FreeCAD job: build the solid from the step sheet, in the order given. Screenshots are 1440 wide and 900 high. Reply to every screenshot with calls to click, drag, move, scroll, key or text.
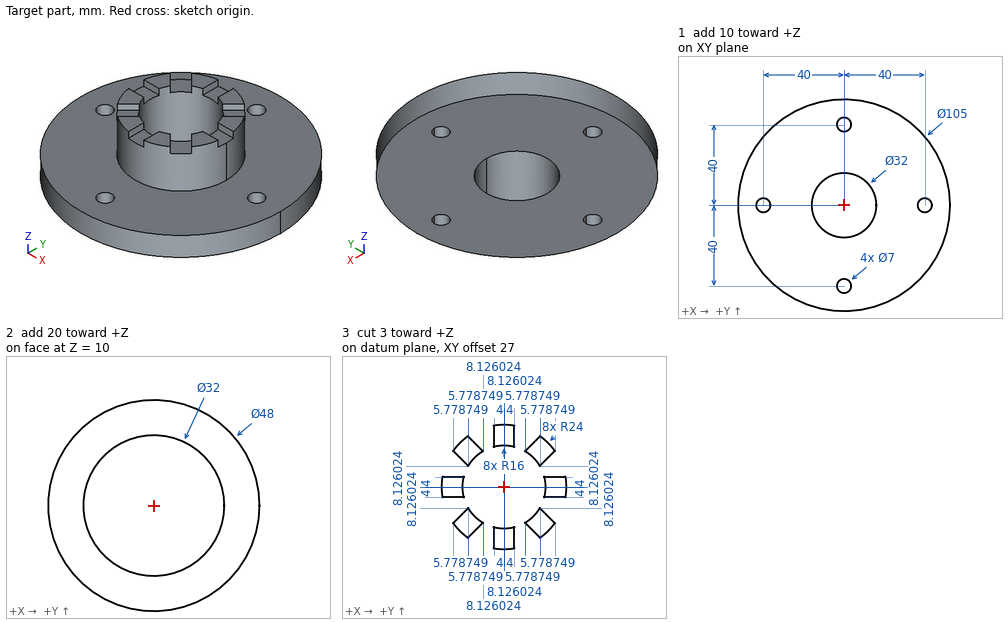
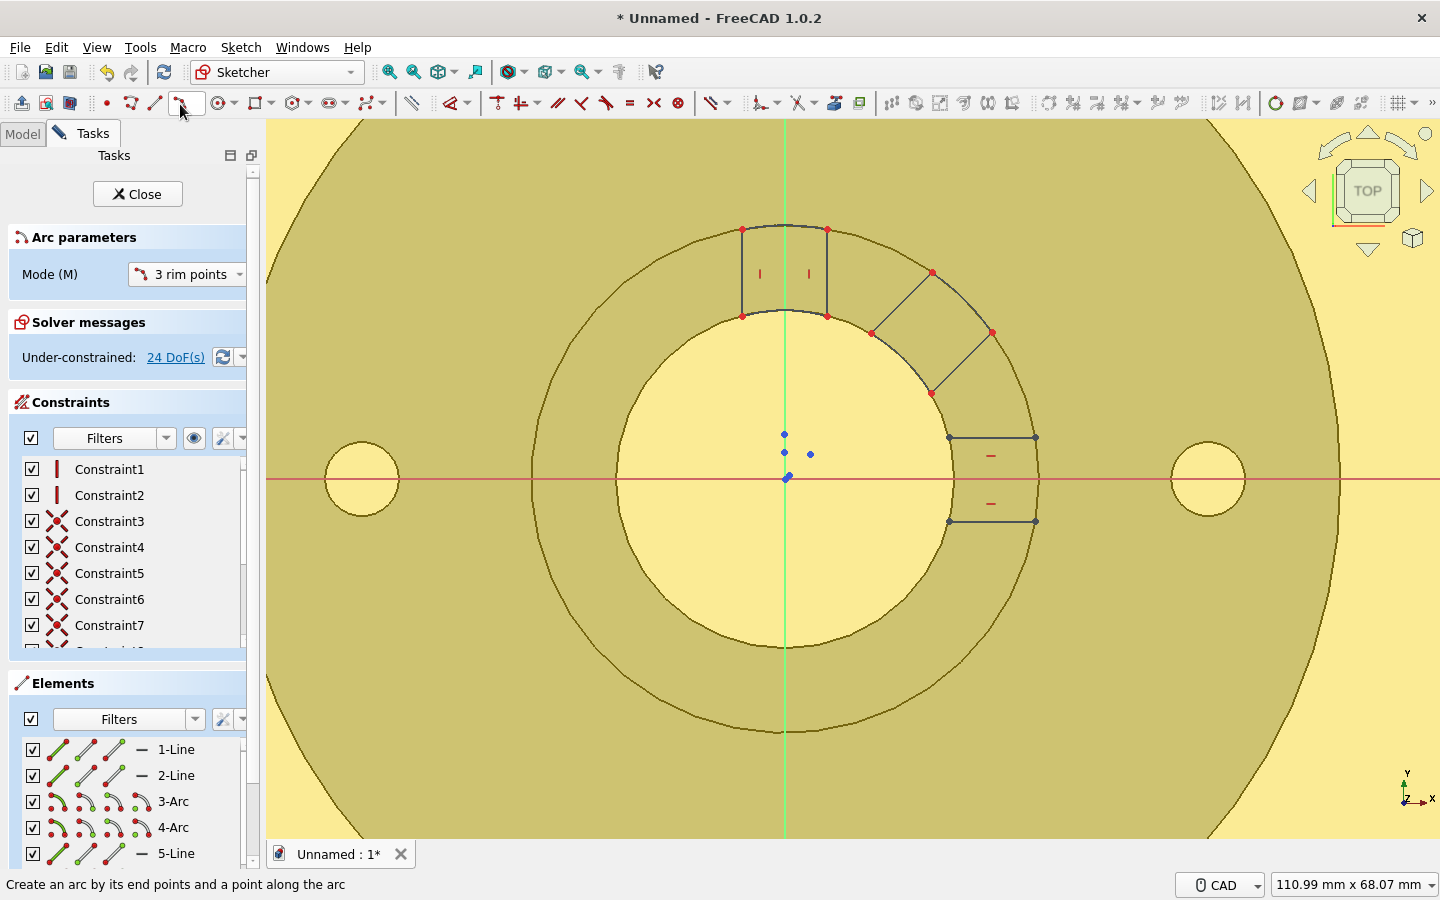
click(949, 438)
click(949, 522)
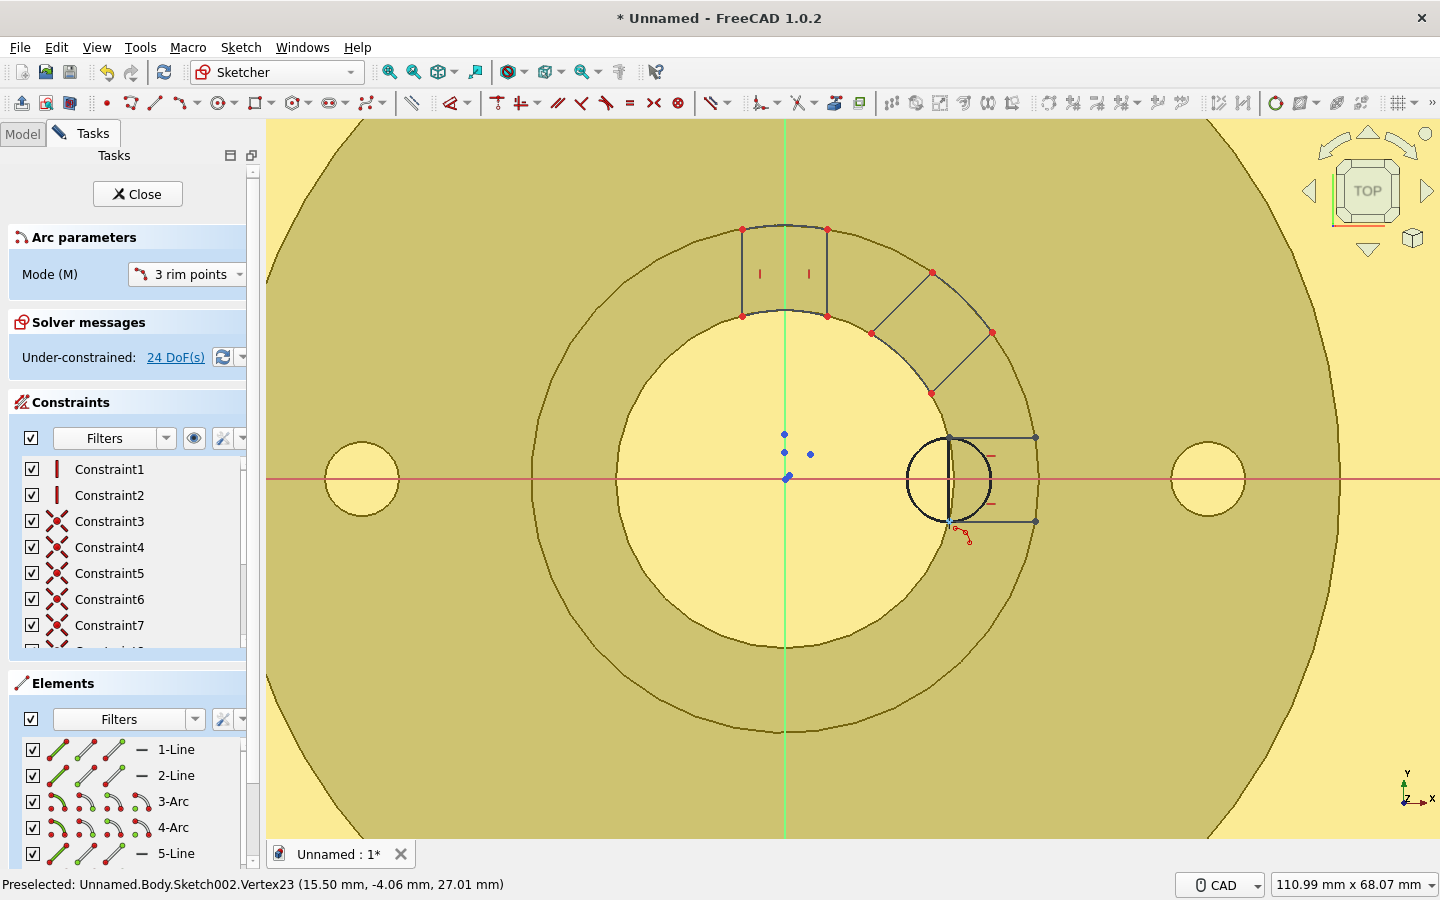
scroll(954, 488, up, 6)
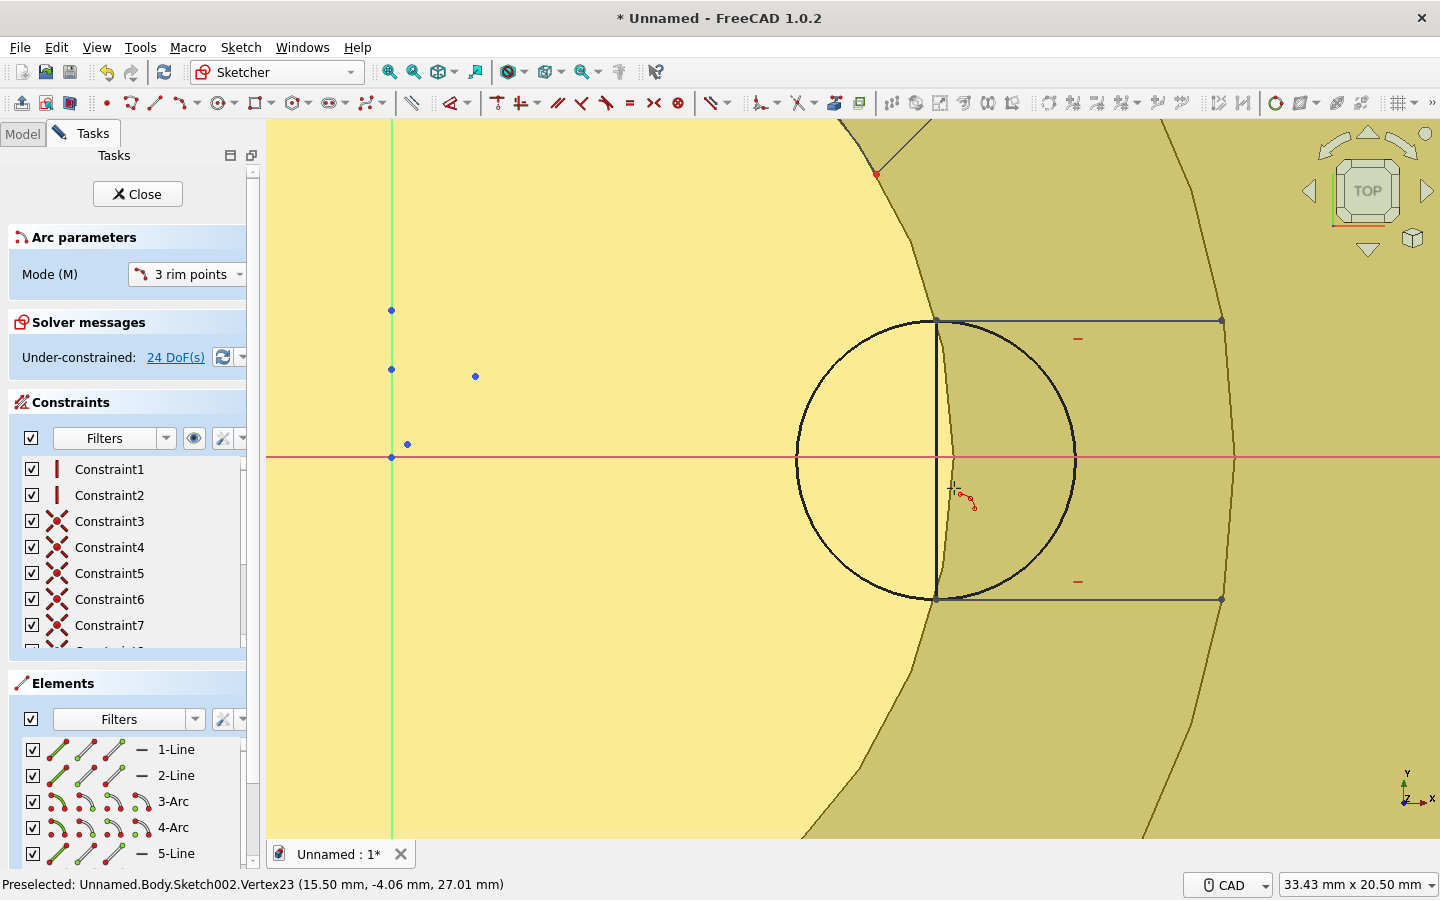
click(953, 486)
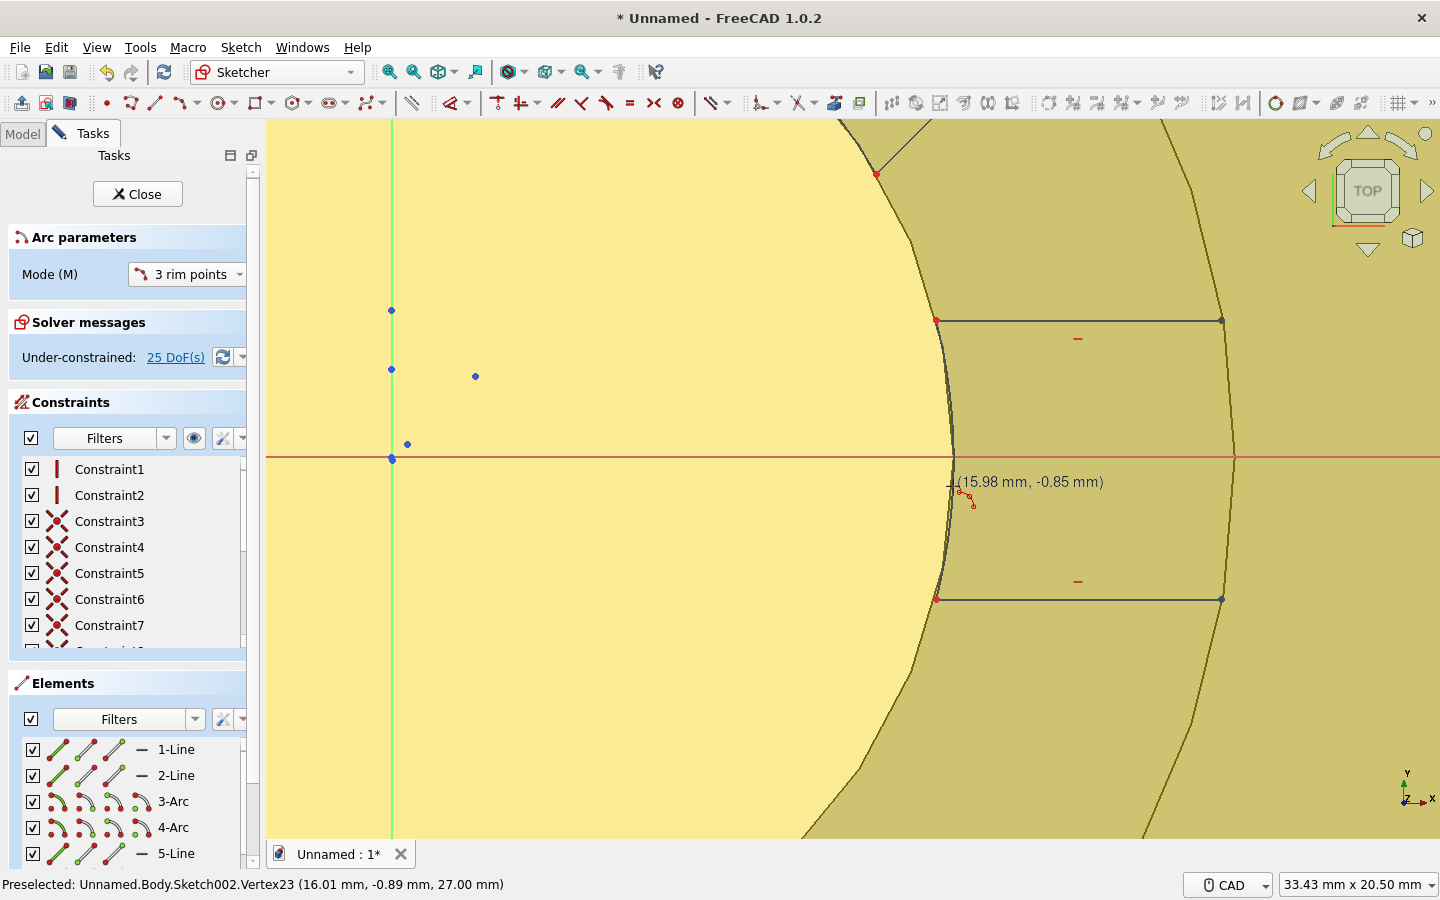
click(1222, 600)
click(1222, 321)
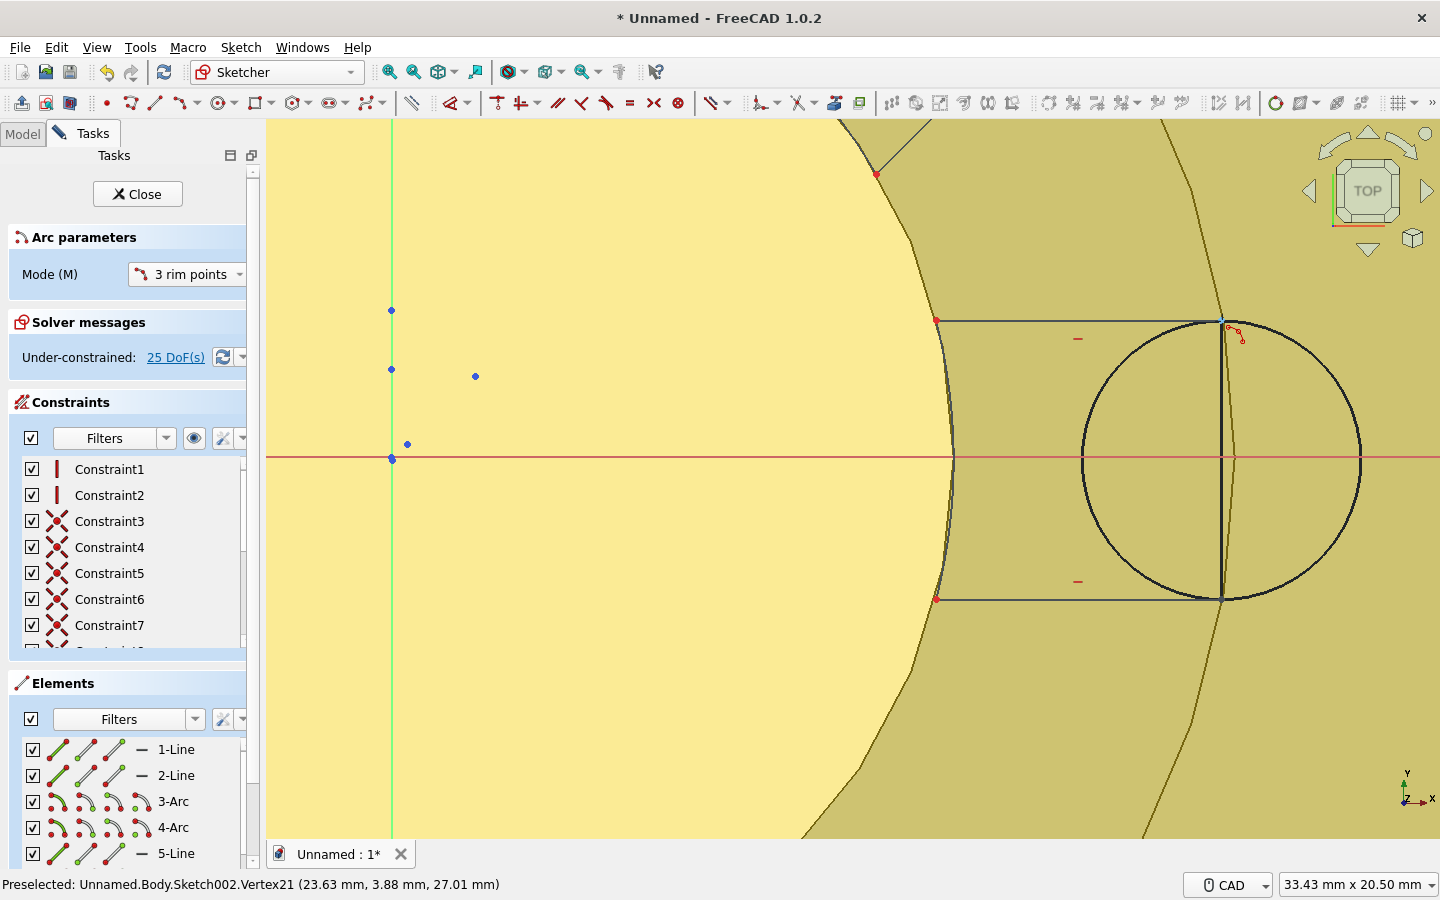
scroll(1234, 485, up, 2)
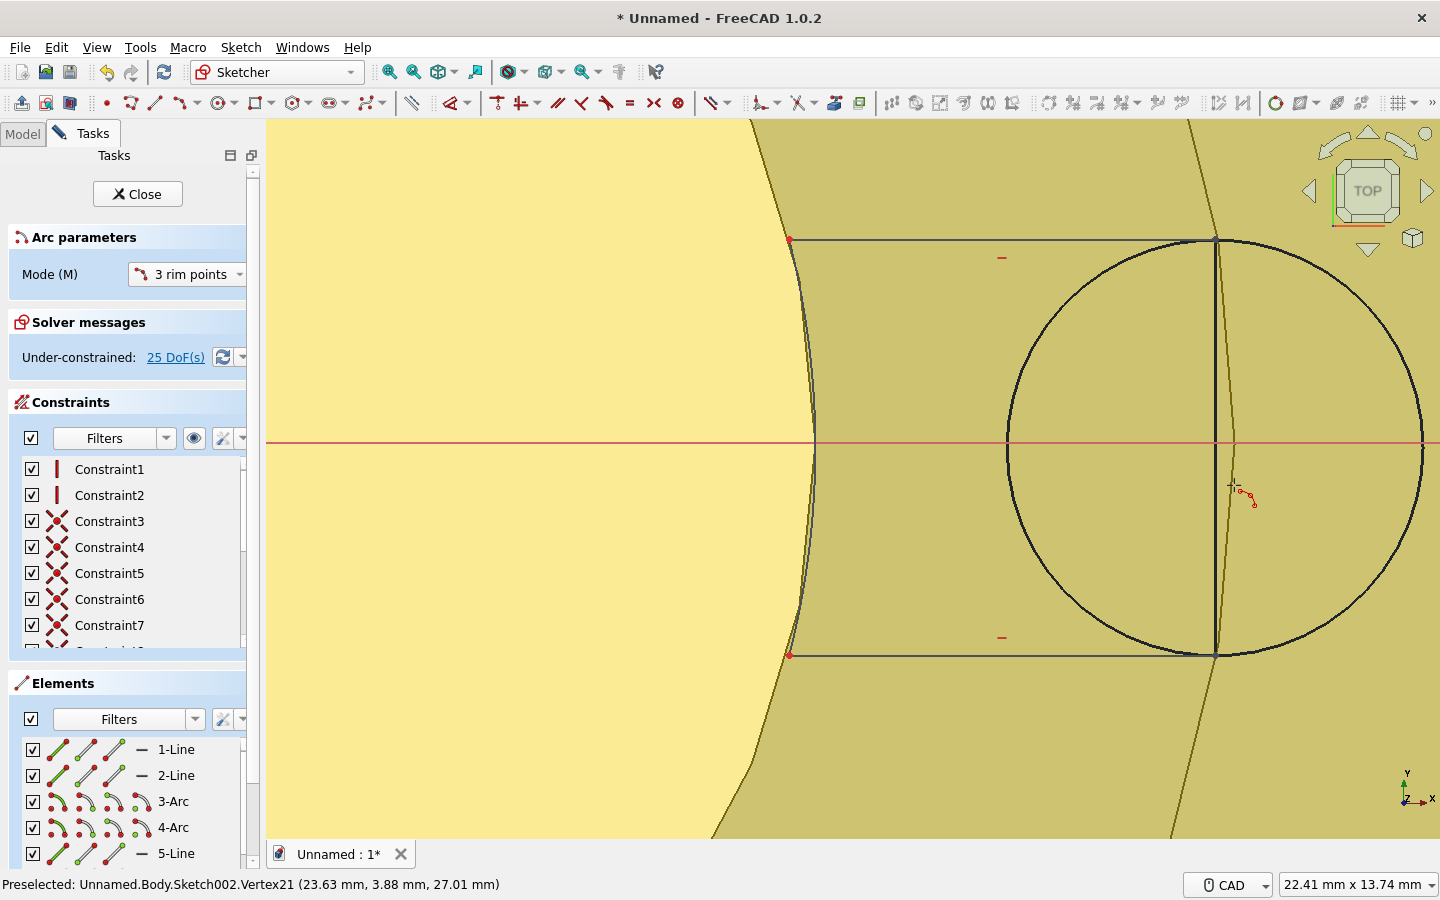
click(1234, 485)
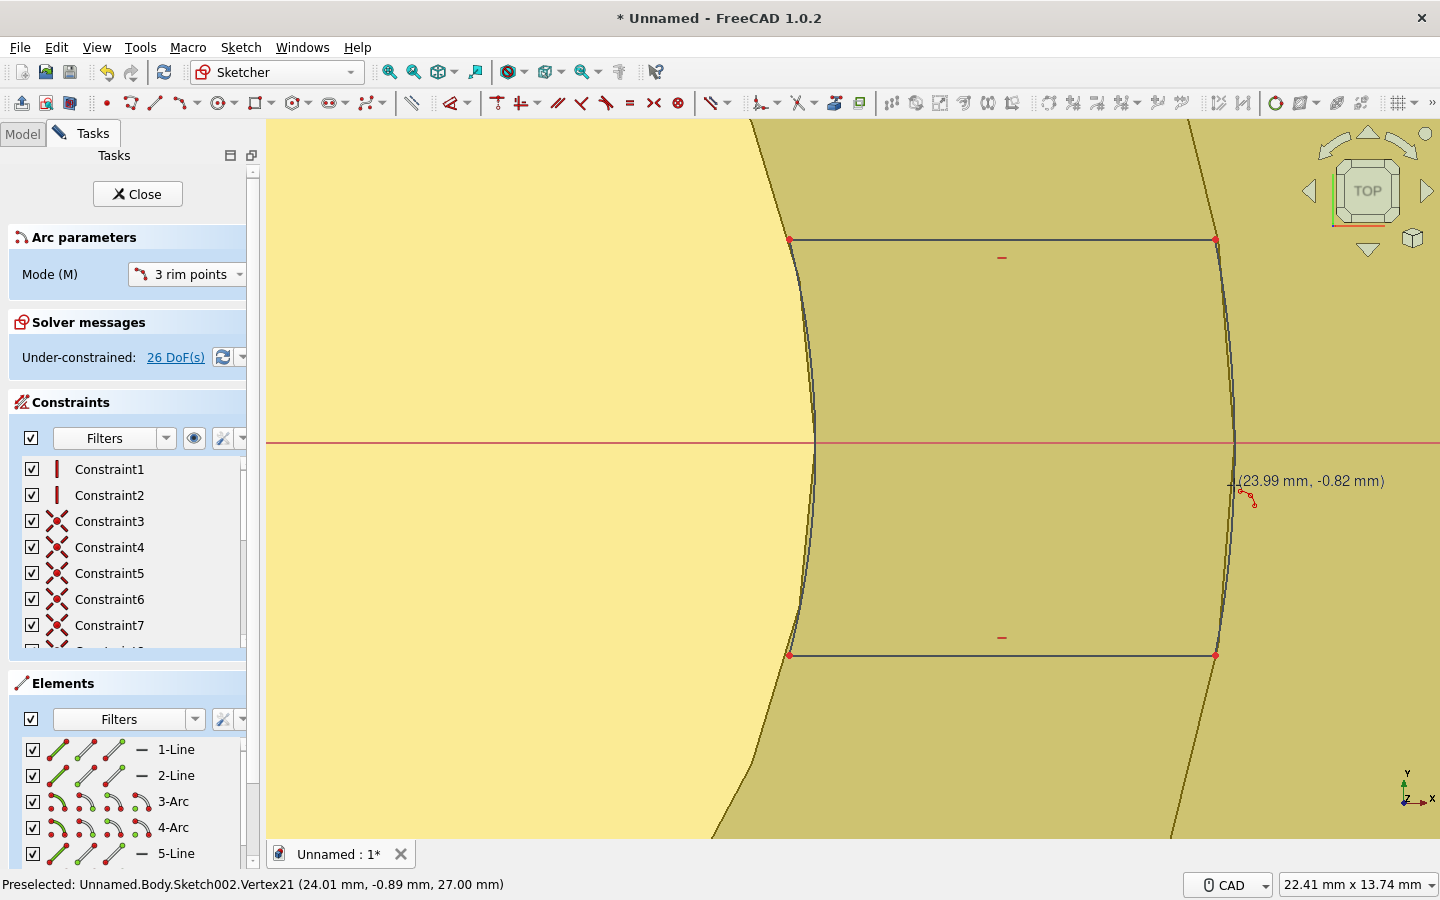
click(156, 104)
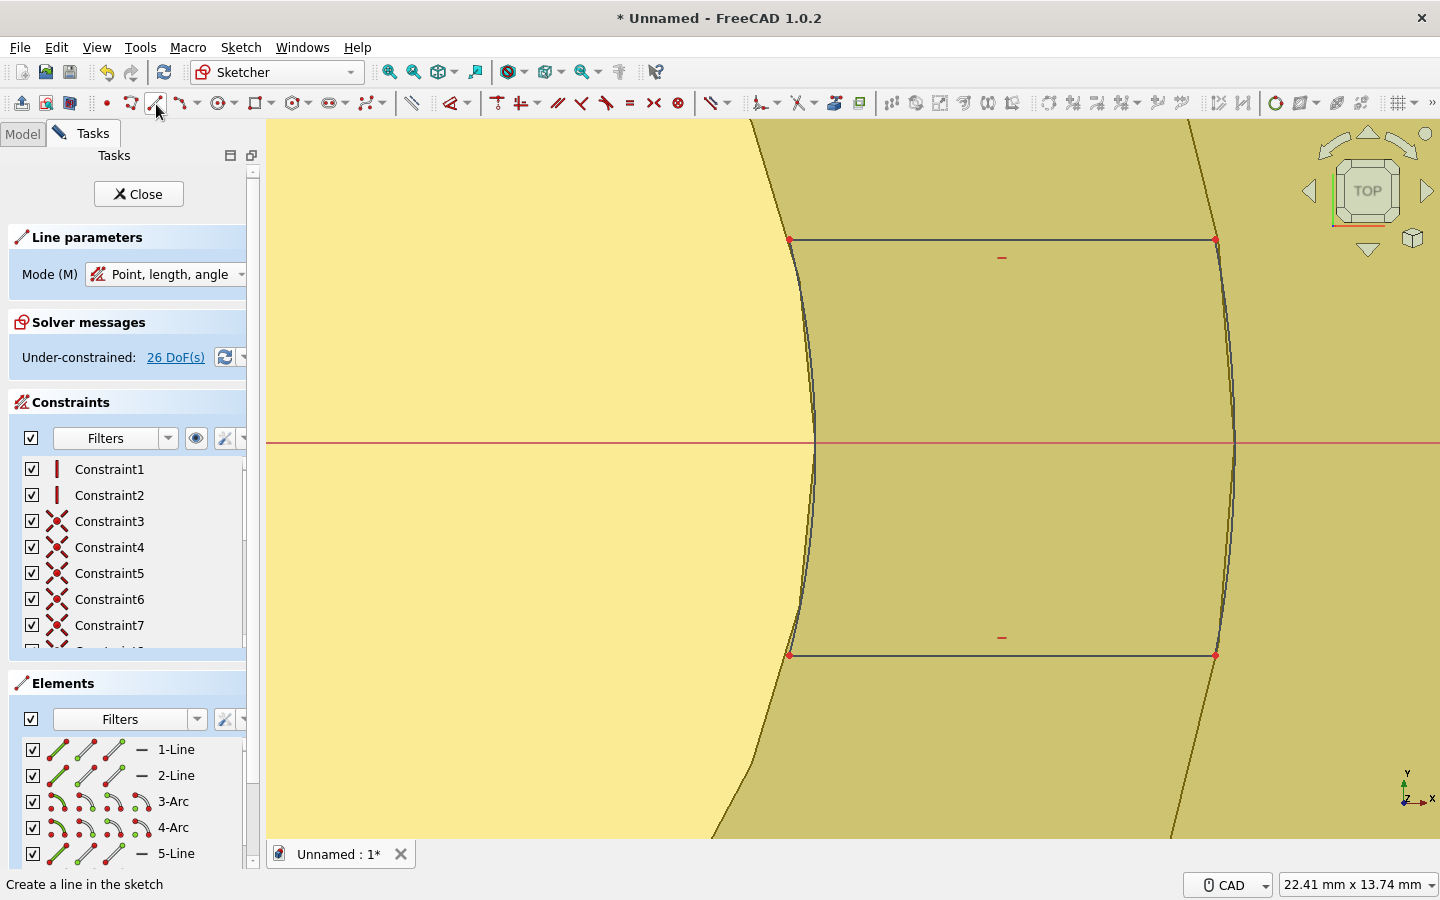
scroll(989, 488, down, 8)